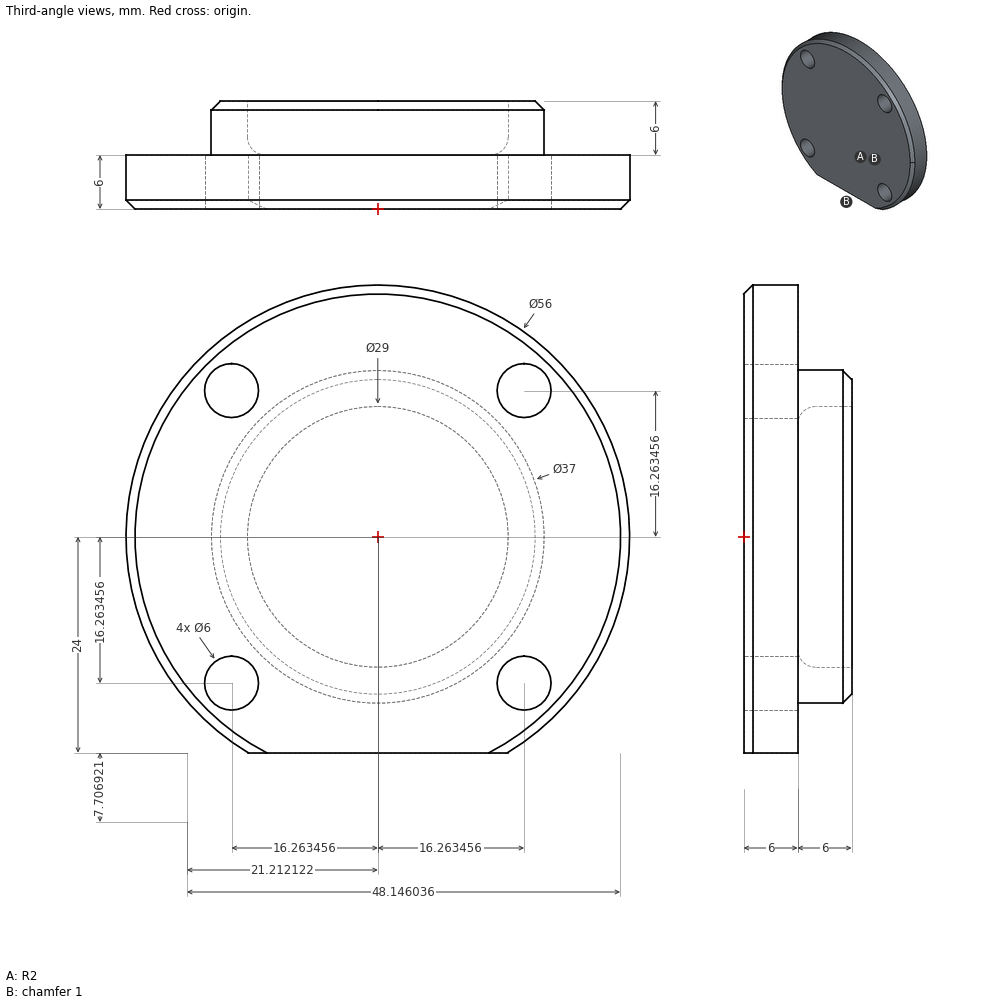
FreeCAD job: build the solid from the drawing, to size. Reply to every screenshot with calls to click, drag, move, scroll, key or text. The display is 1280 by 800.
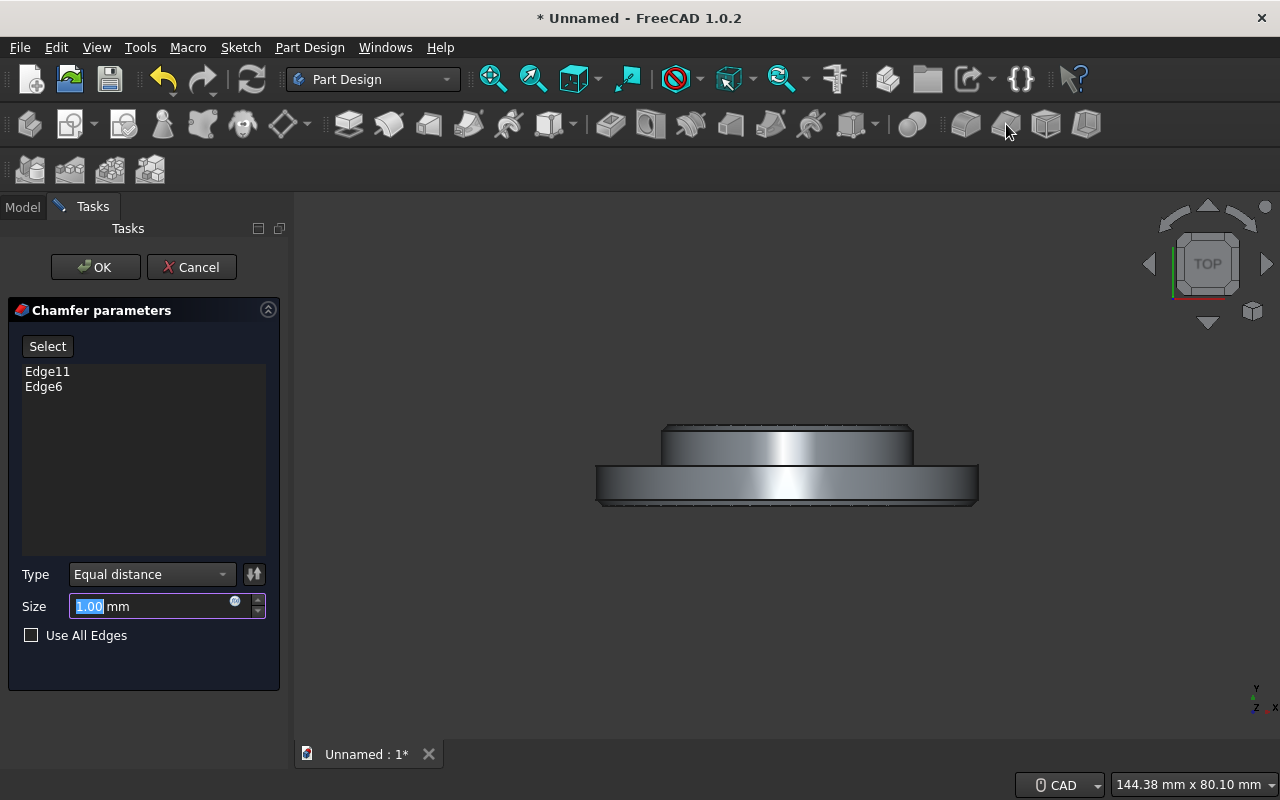
text(1)
key(Tab)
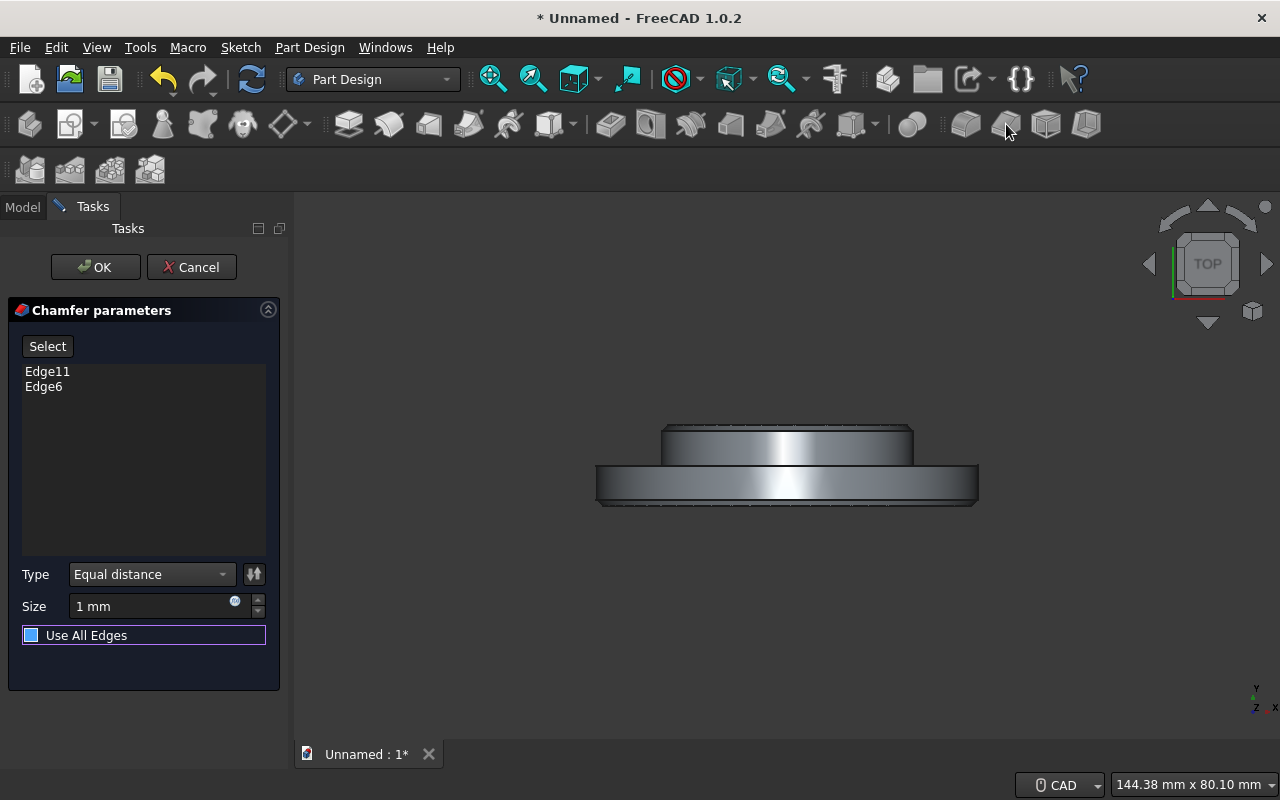
click(96, 267)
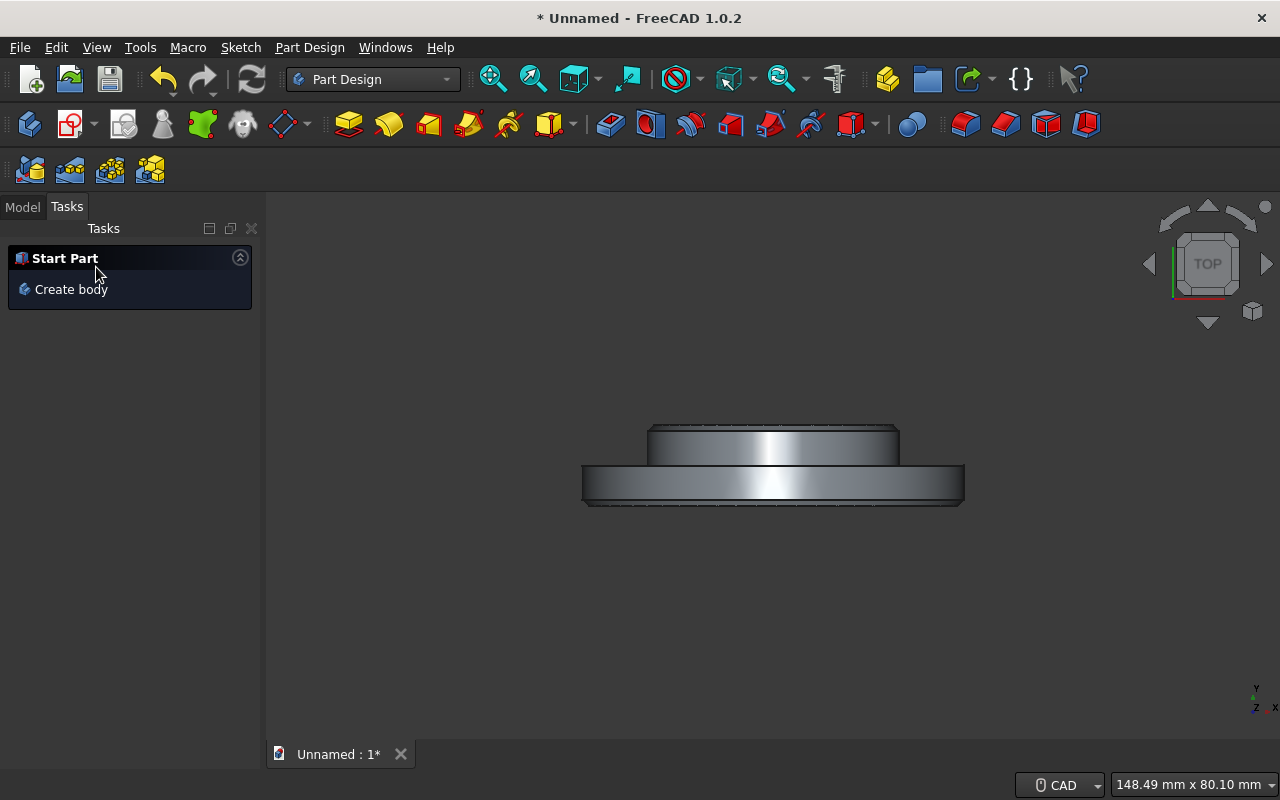
key(v)
key(f)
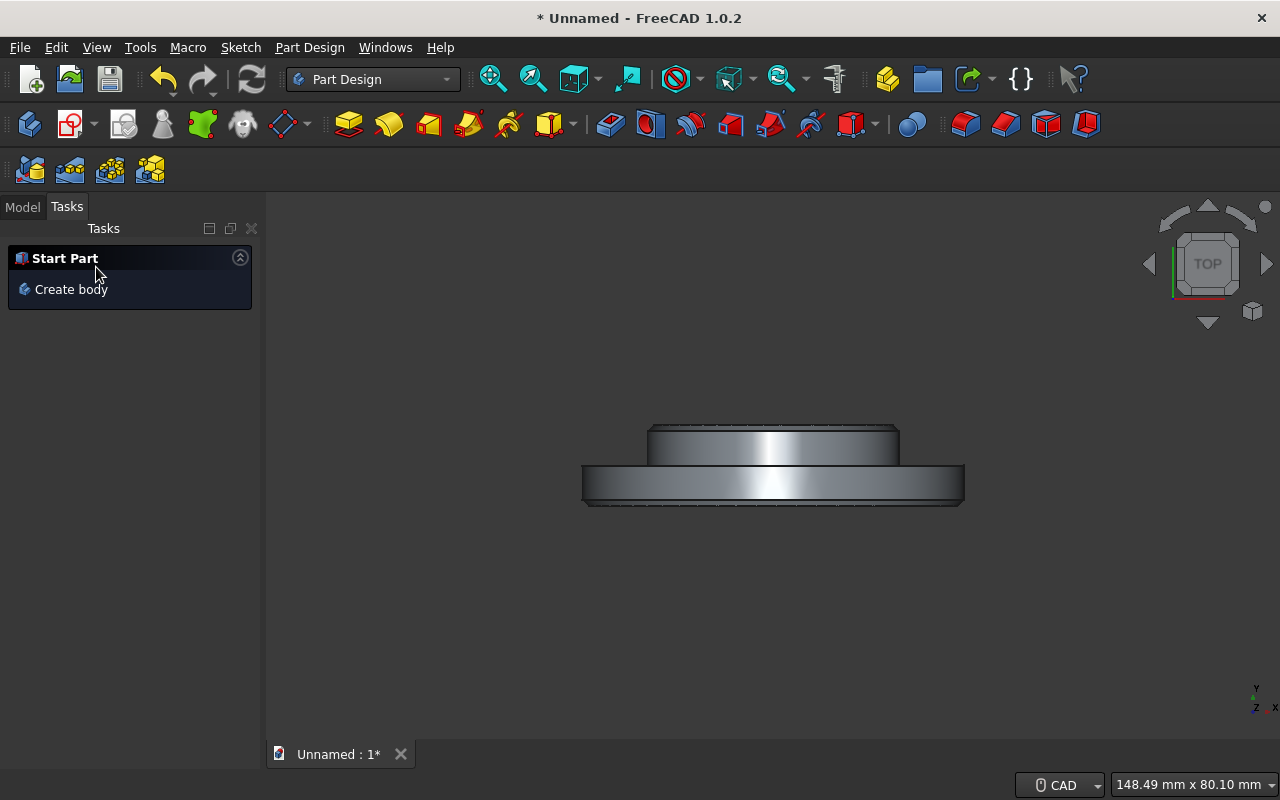
key(4)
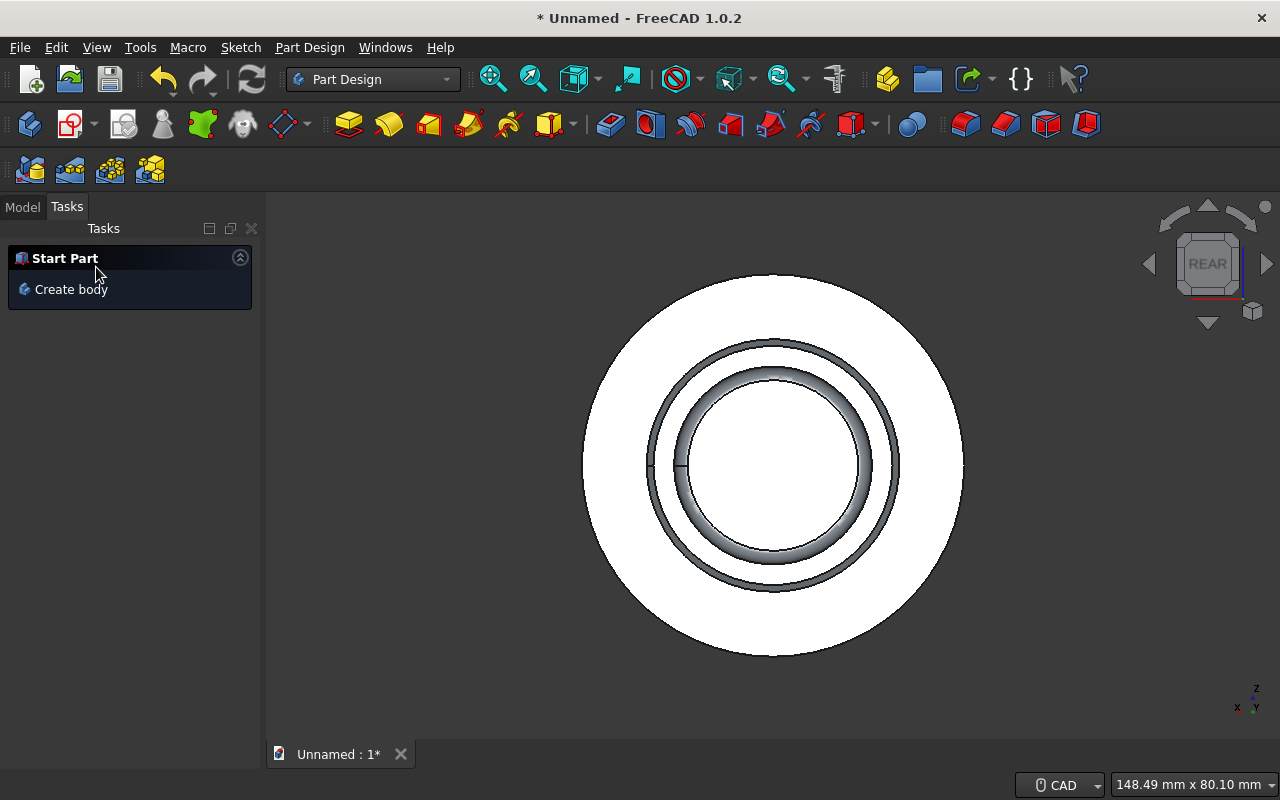
click(664, 574)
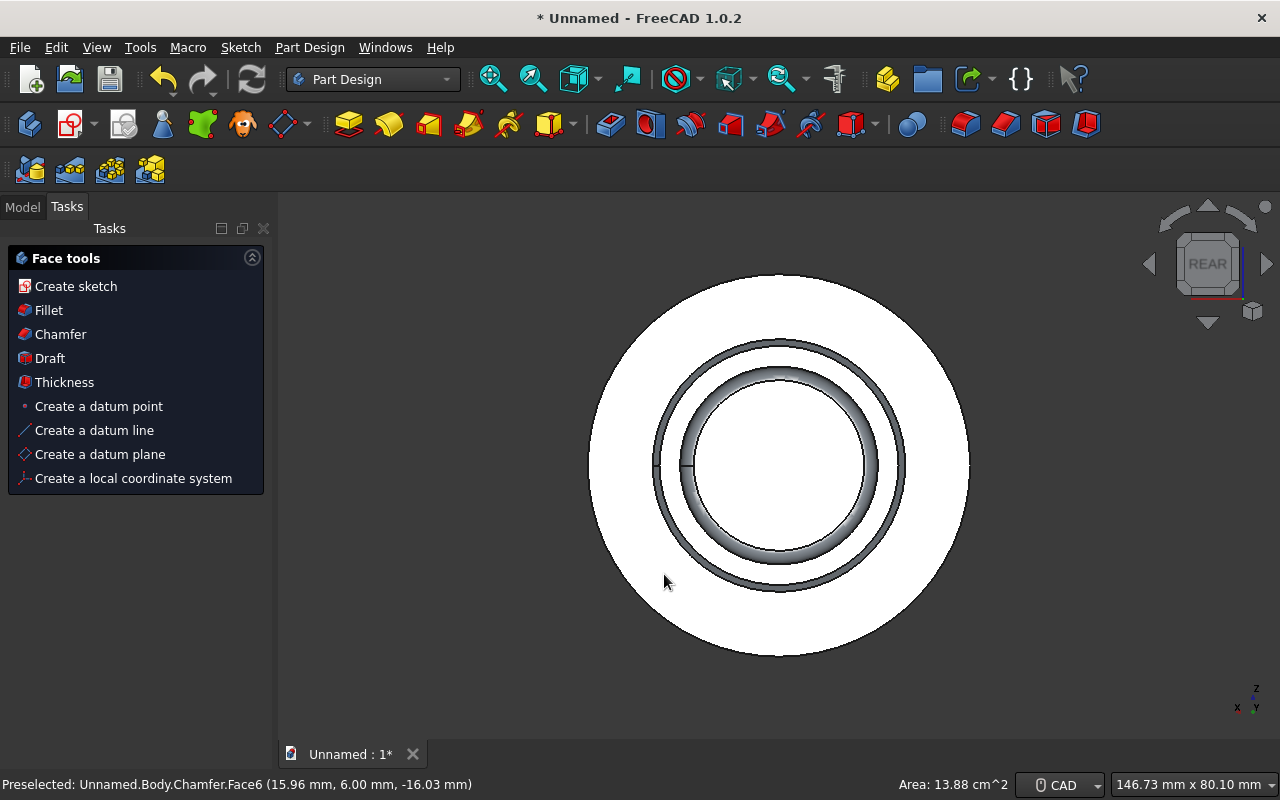
click(70, 124)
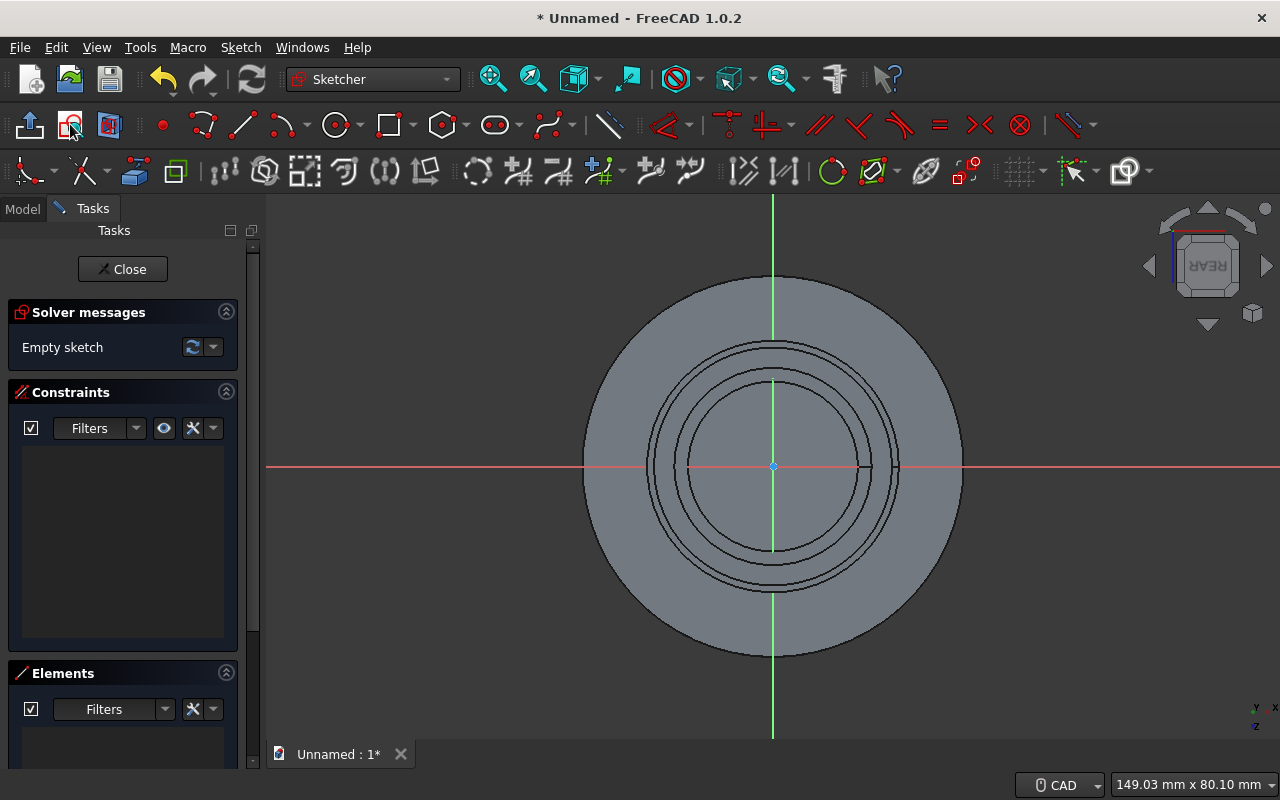
key(q)
key(s)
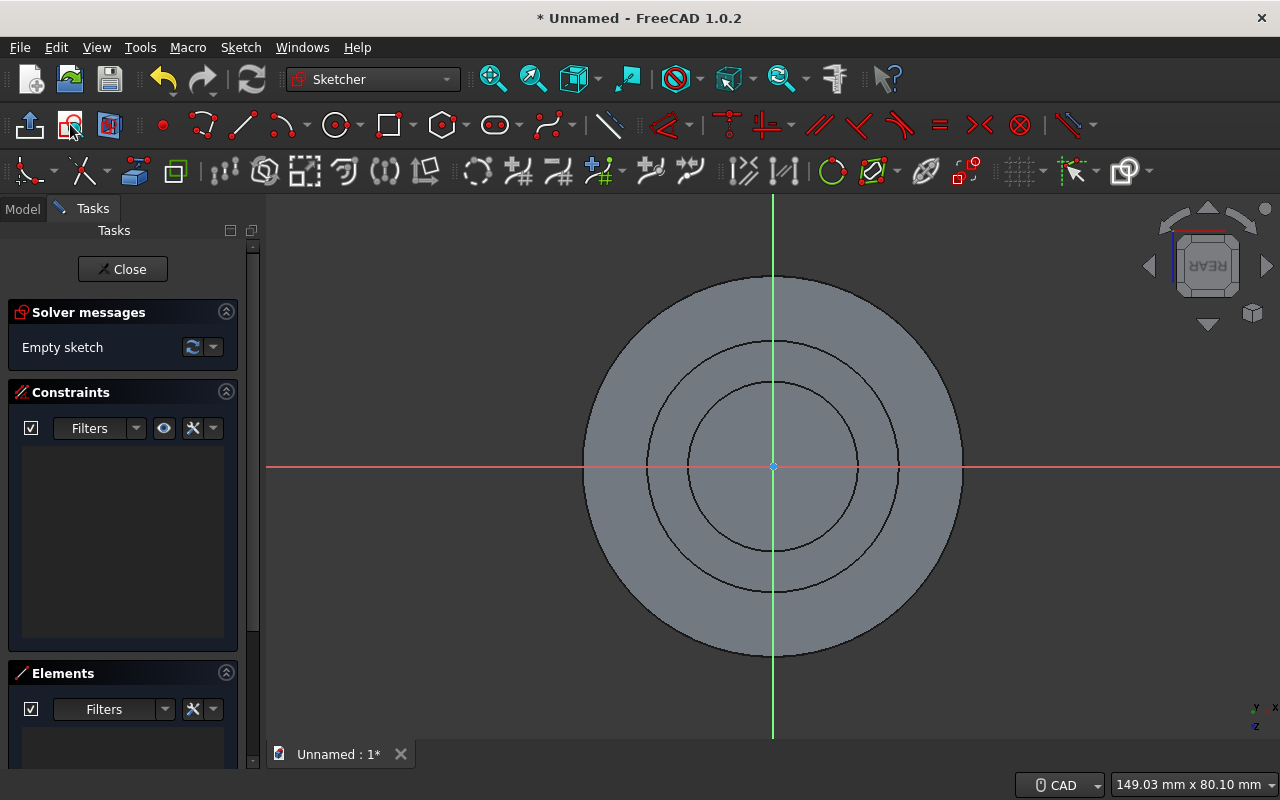
key(g)
key(c)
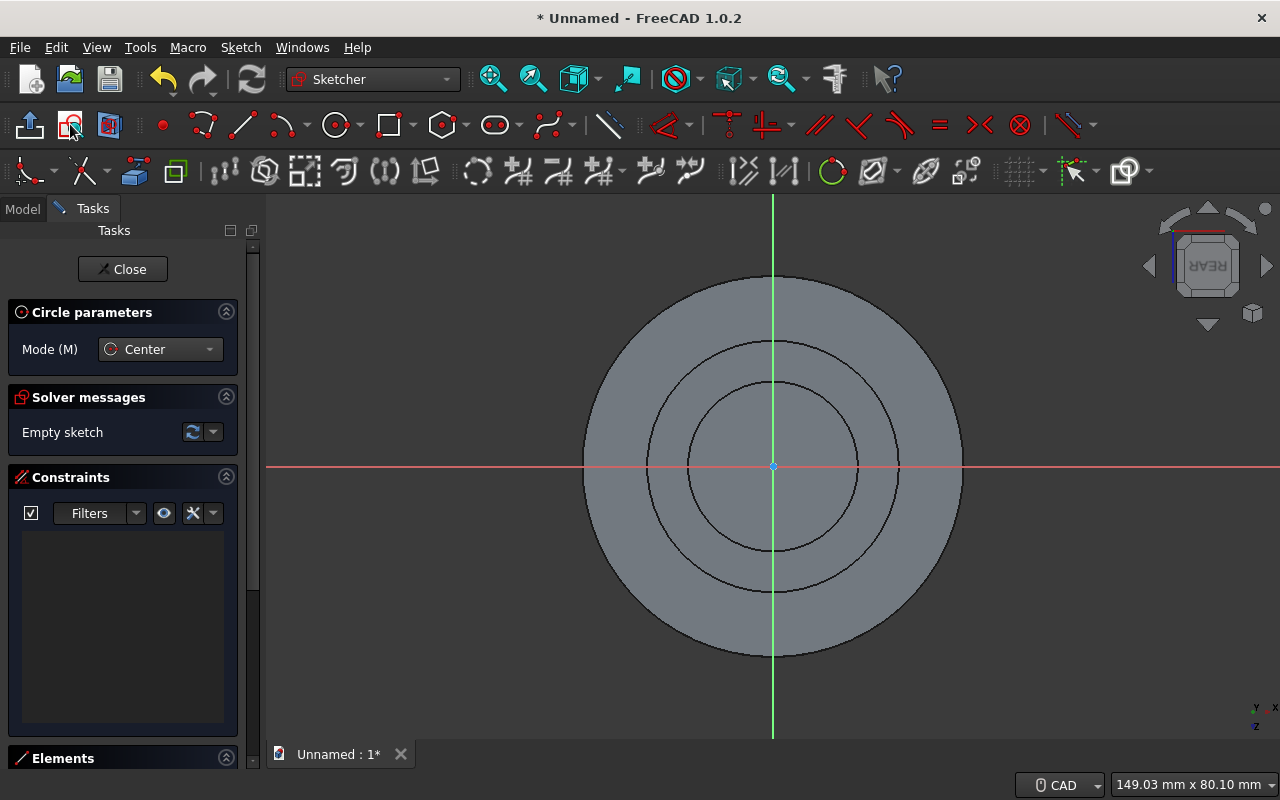
click(662, 356)
click(677, 341)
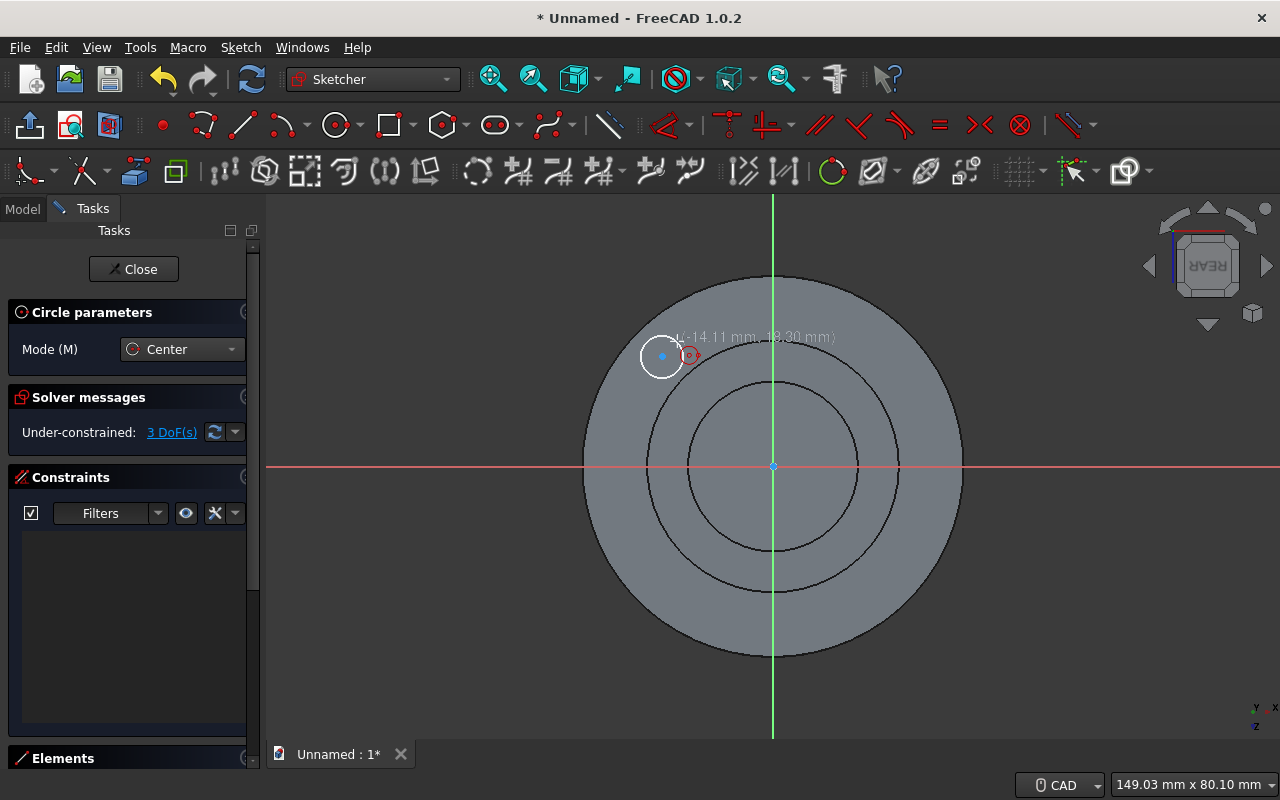
click(884, 356)
click(898, 341)